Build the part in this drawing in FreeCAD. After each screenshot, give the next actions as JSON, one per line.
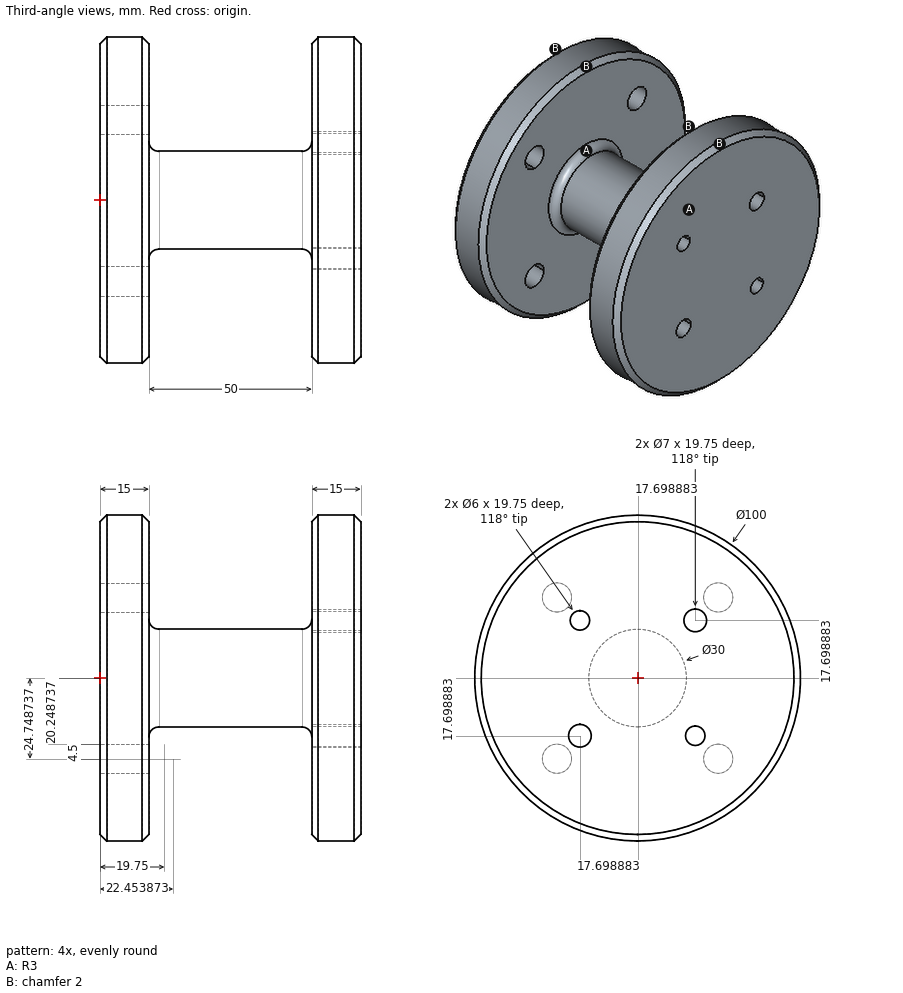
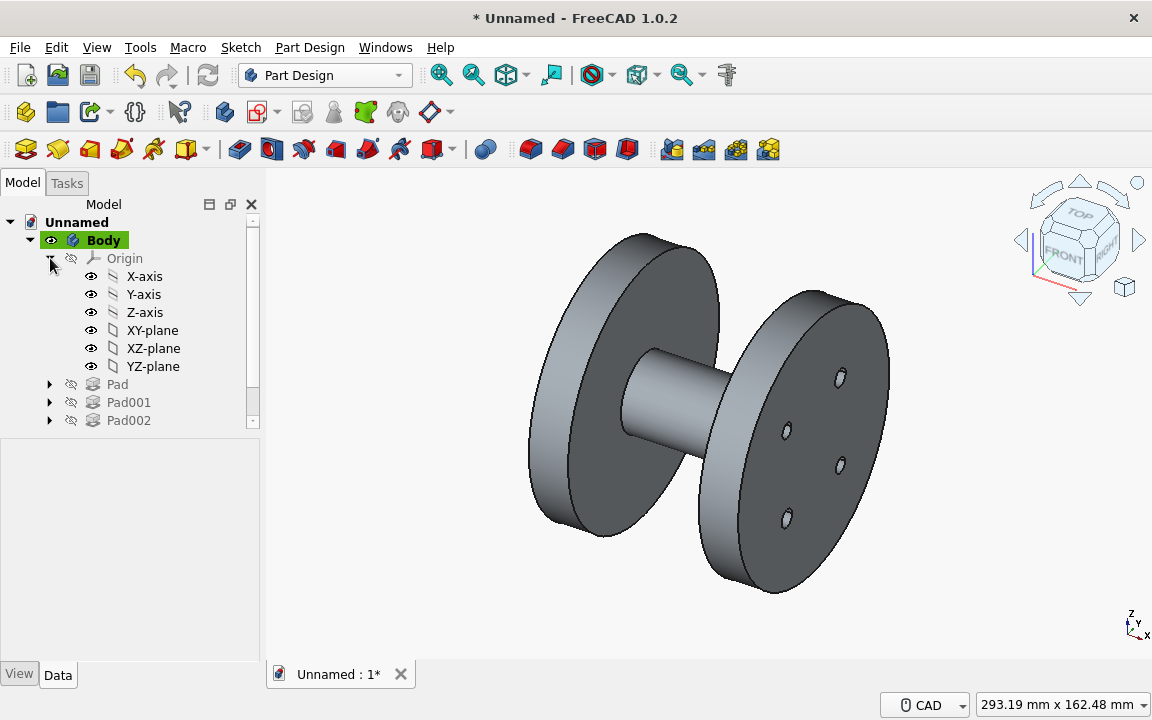
{"action": "left_click", "coordinate": [136, 348]}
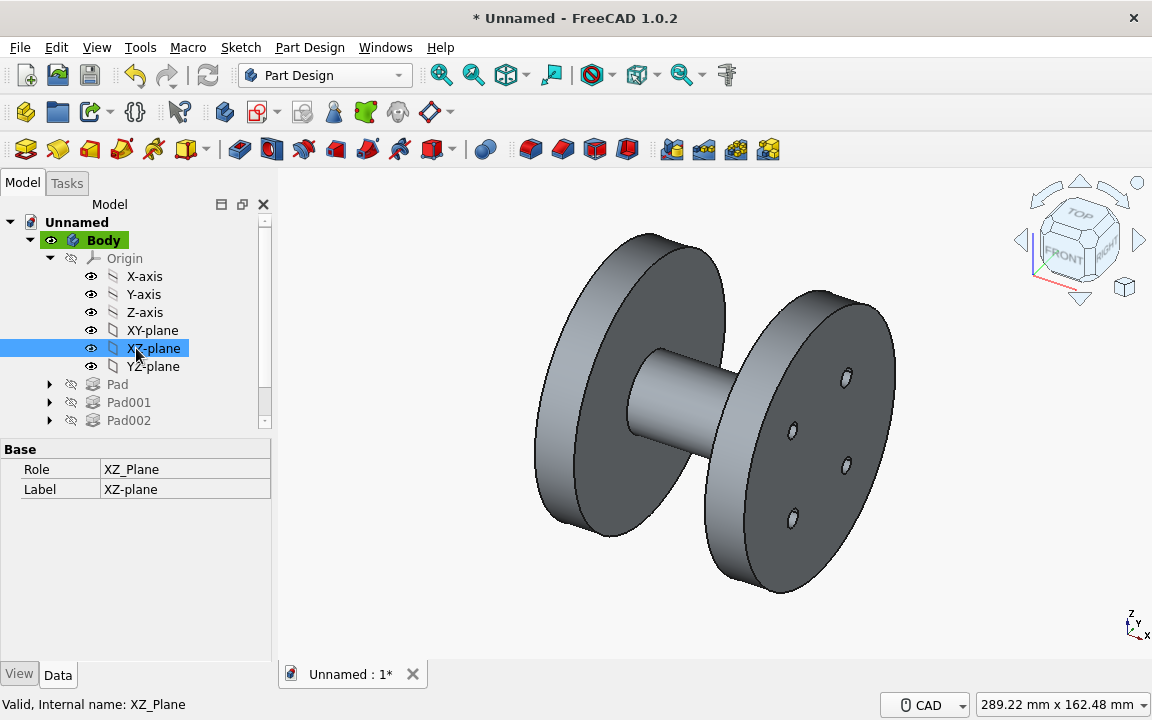
{"action": "left_click", "coordinate": [430, 112]}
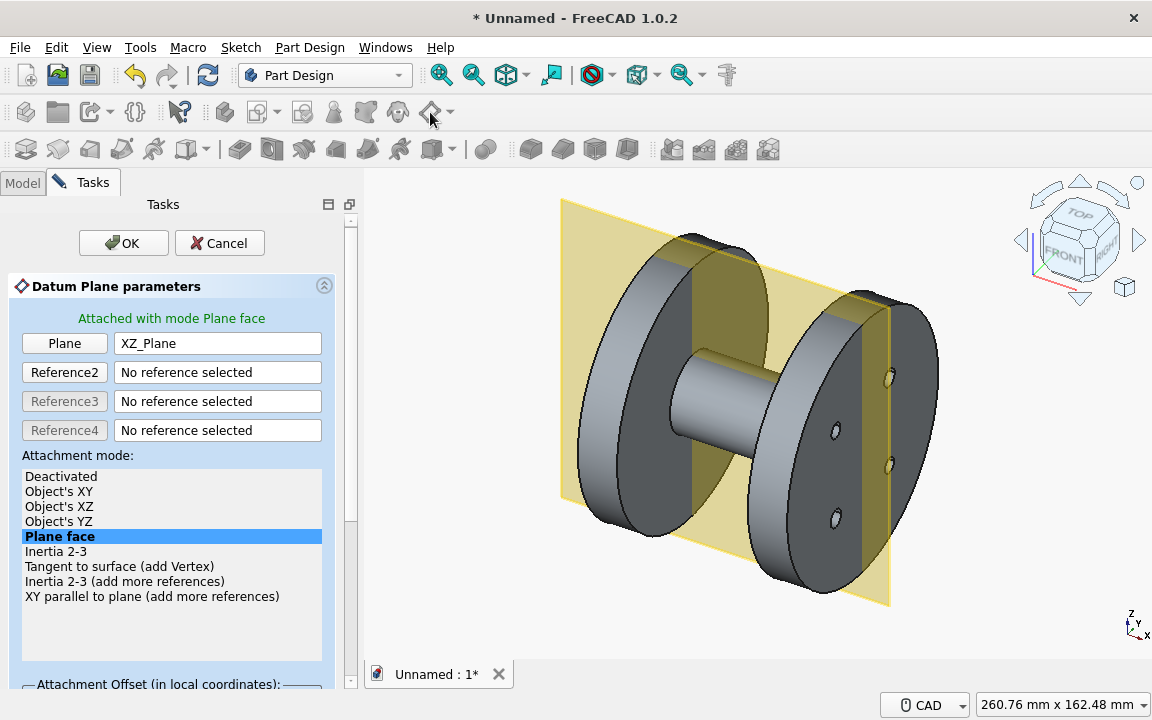
{"action": "scroll", "coordinate": [351, 451], "scroll_direction": "down", "scroll_amount": 3}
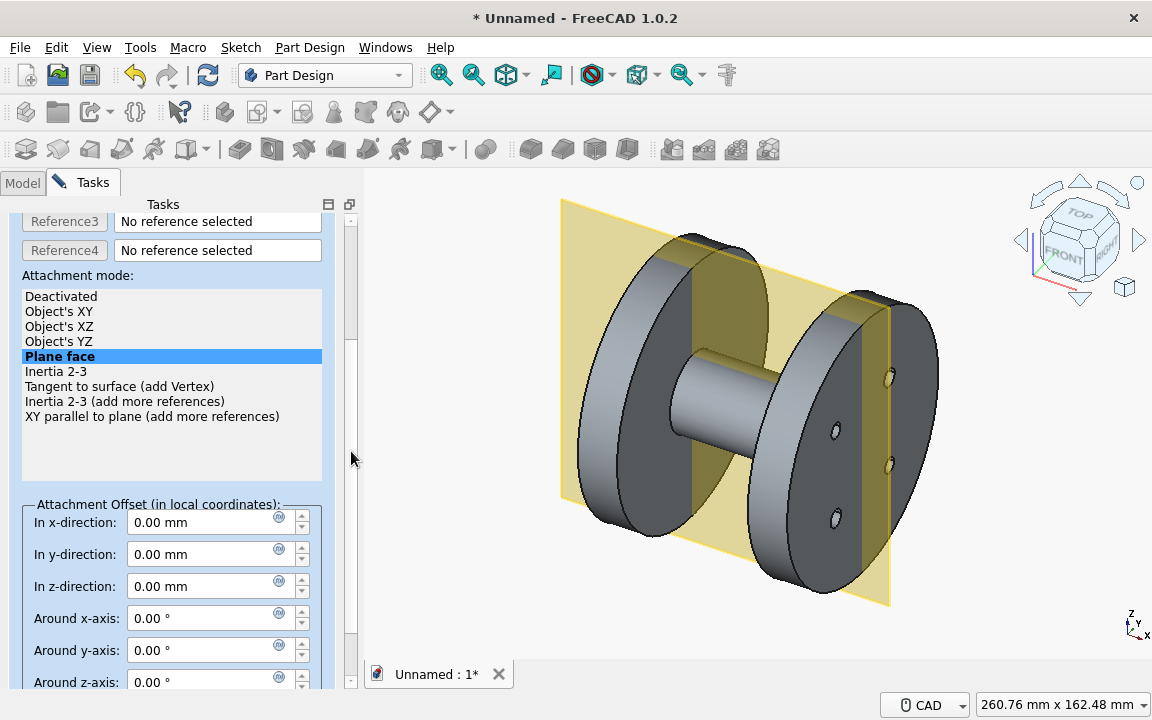
{"action": "triple_click", "coordinate": [210, 586]}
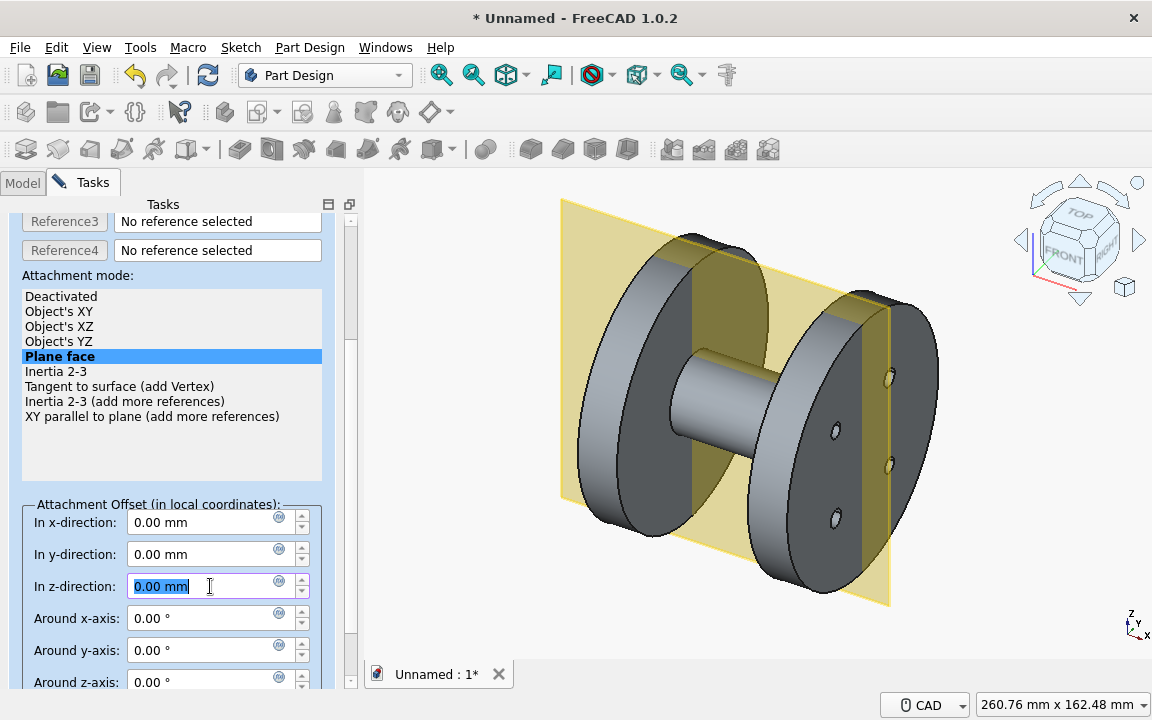
{"action": "type", "text": "-24.748737"}
{"action": "key", "text": "Tab"}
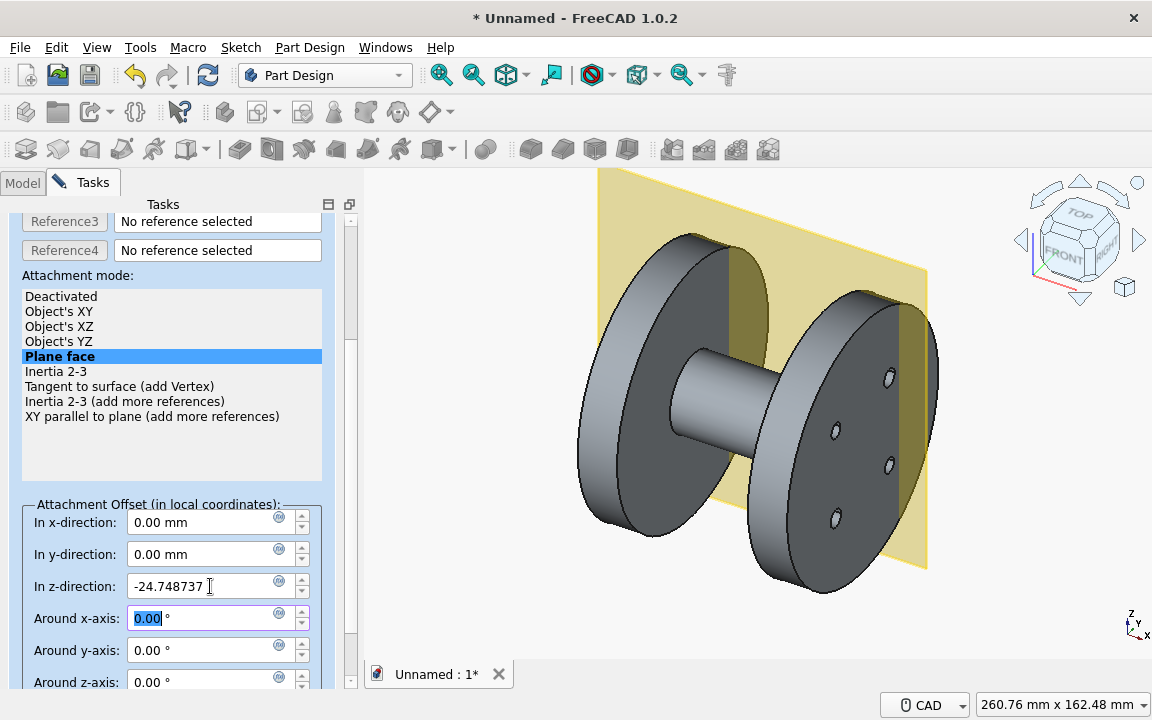
{"action": "scroll", "coordinate": [351, 451], "scroll_direction": "up", "scroll_amount": 4}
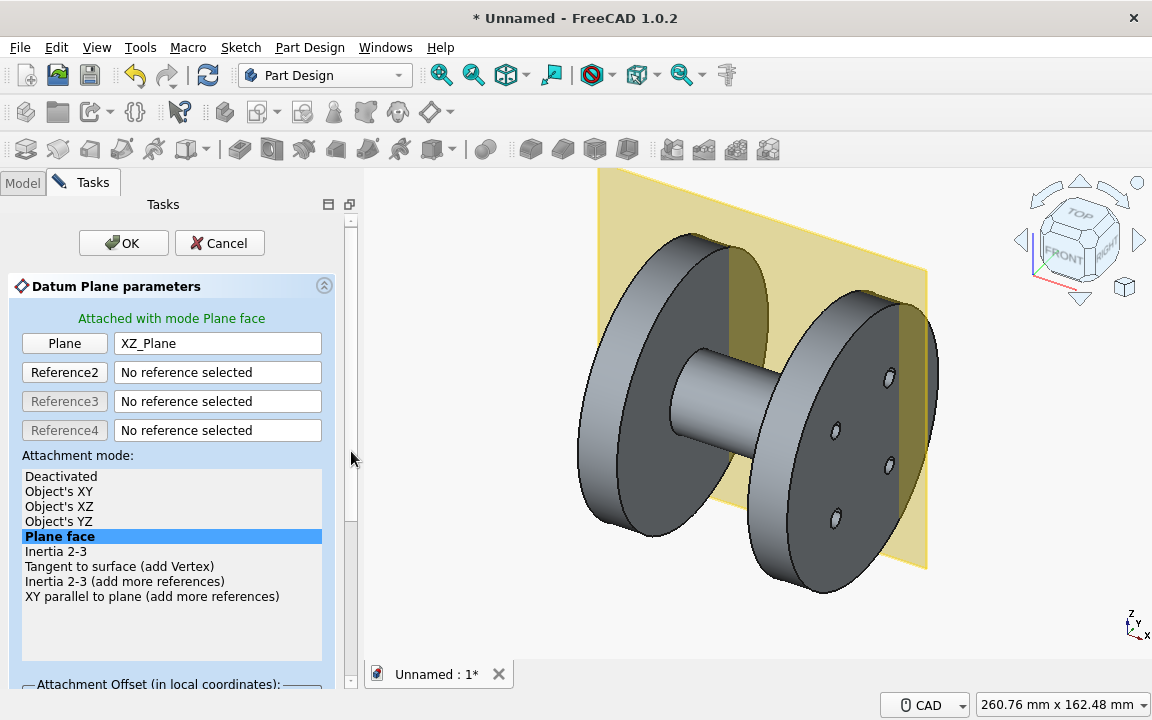
{"action": "left_click", "coordinate": [124, 243]}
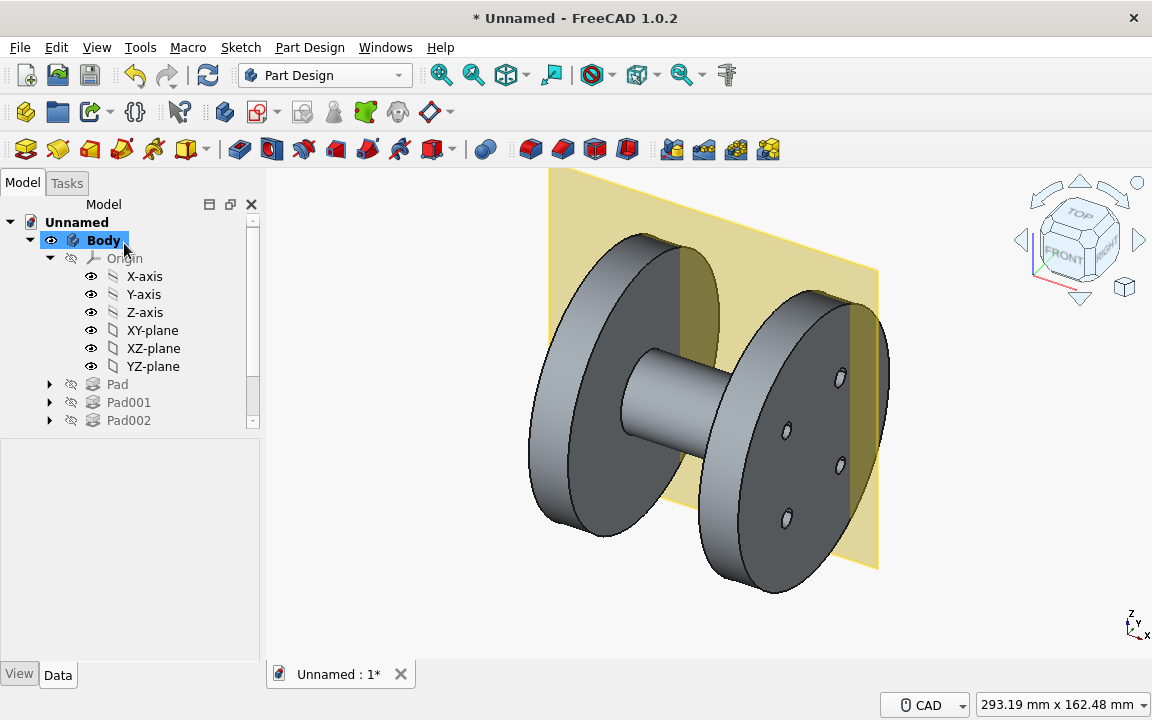
{"action": "scroll", "coordinate": [100, 326], "scroll_direction": "down", "scroll_amount": 3}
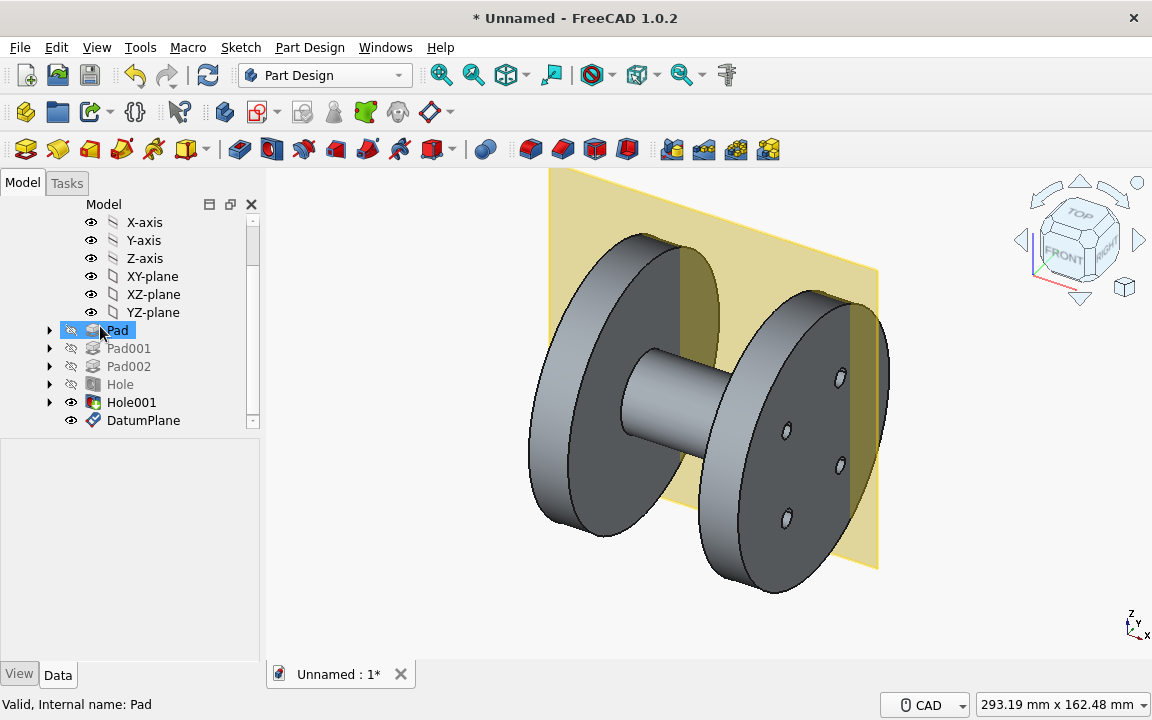
{"action": "left_click", "coordinate": [116, 420]}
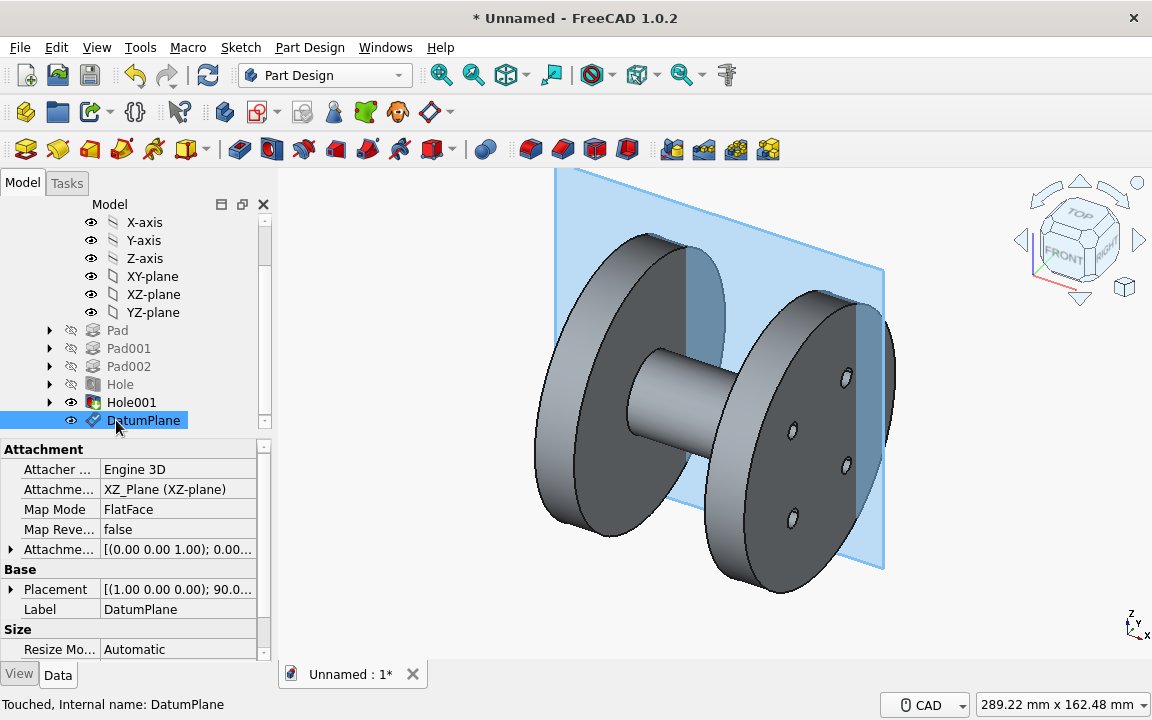
{"action": "left_click", "coordinate": [258, 112]}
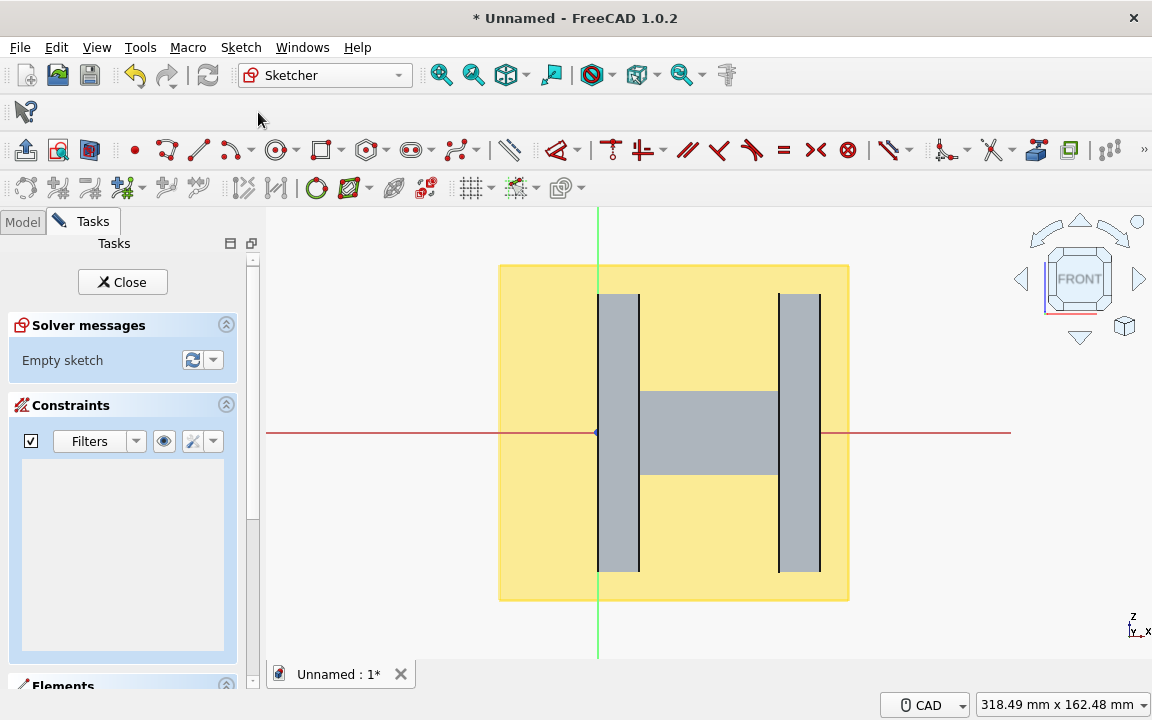
{"action": "left_click", "coordinate": [90, 150]}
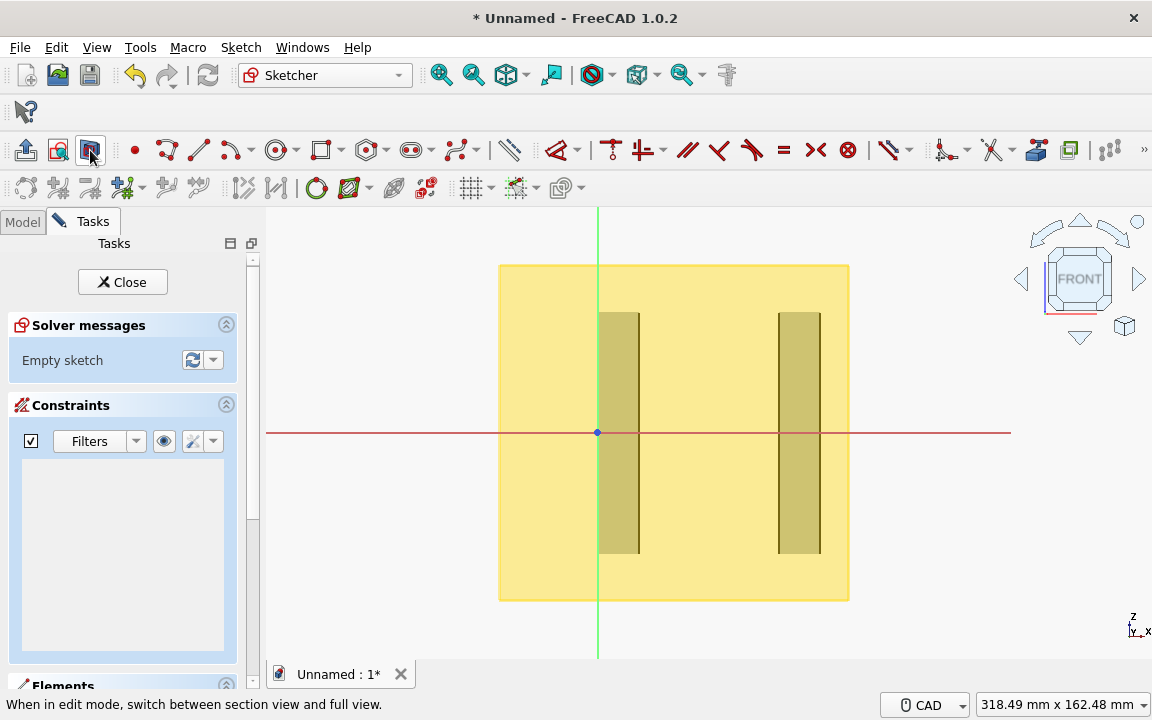
{"action": "scroll", "coordinate": [642, 479], "scroll_direction": "up", "scroll_amount": 7}